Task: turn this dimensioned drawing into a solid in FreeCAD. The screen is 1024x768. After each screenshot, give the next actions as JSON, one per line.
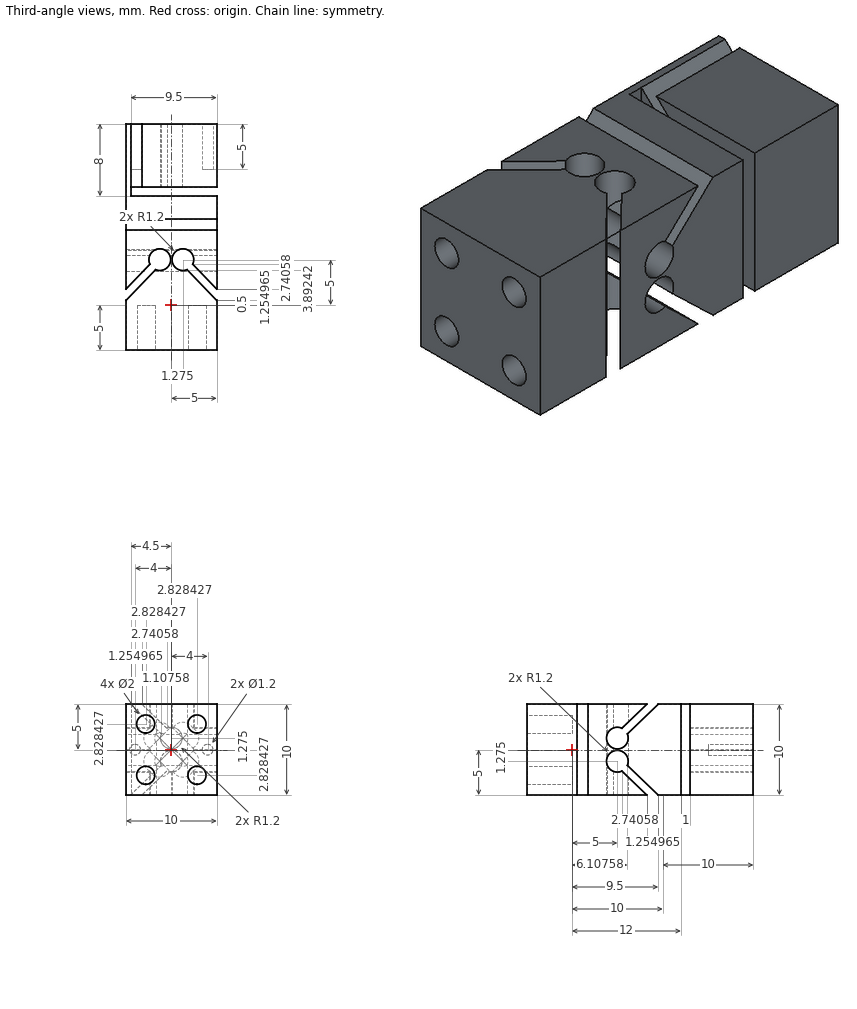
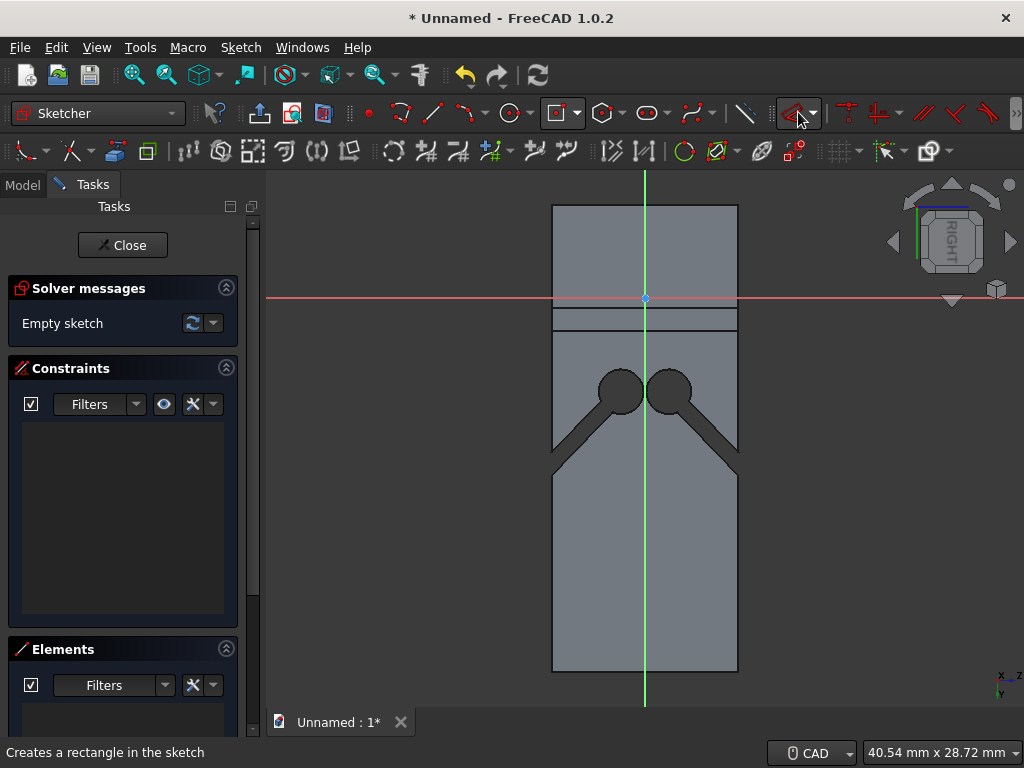
{"action": "scroll", "coordinate": [784, 382], "scroll_direction": "up", "scroll_amount": 2}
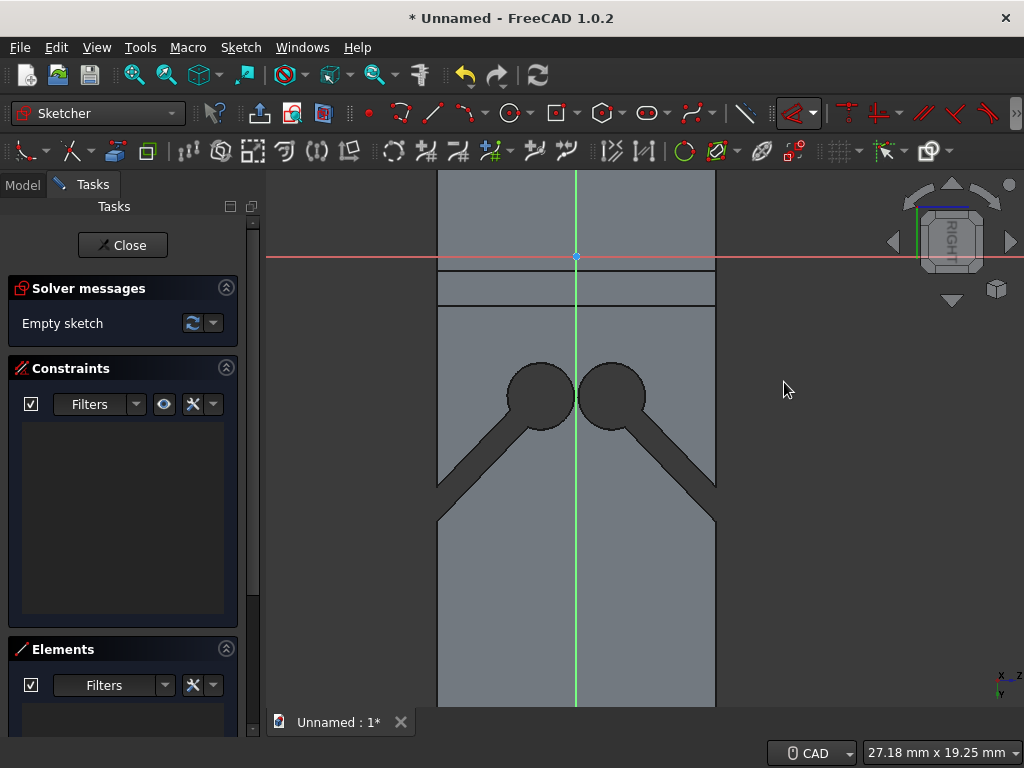
{"action": "left_click", "coordinate": [580, 114]}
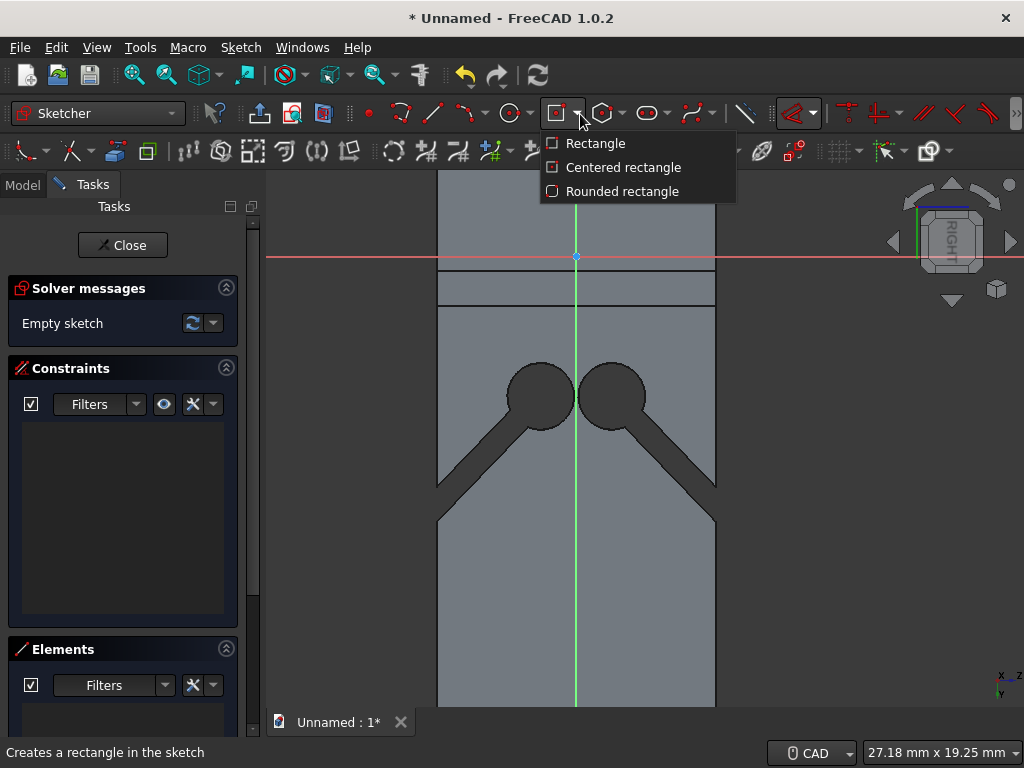
{"action": "left_click", "coordinate": [638, 143]}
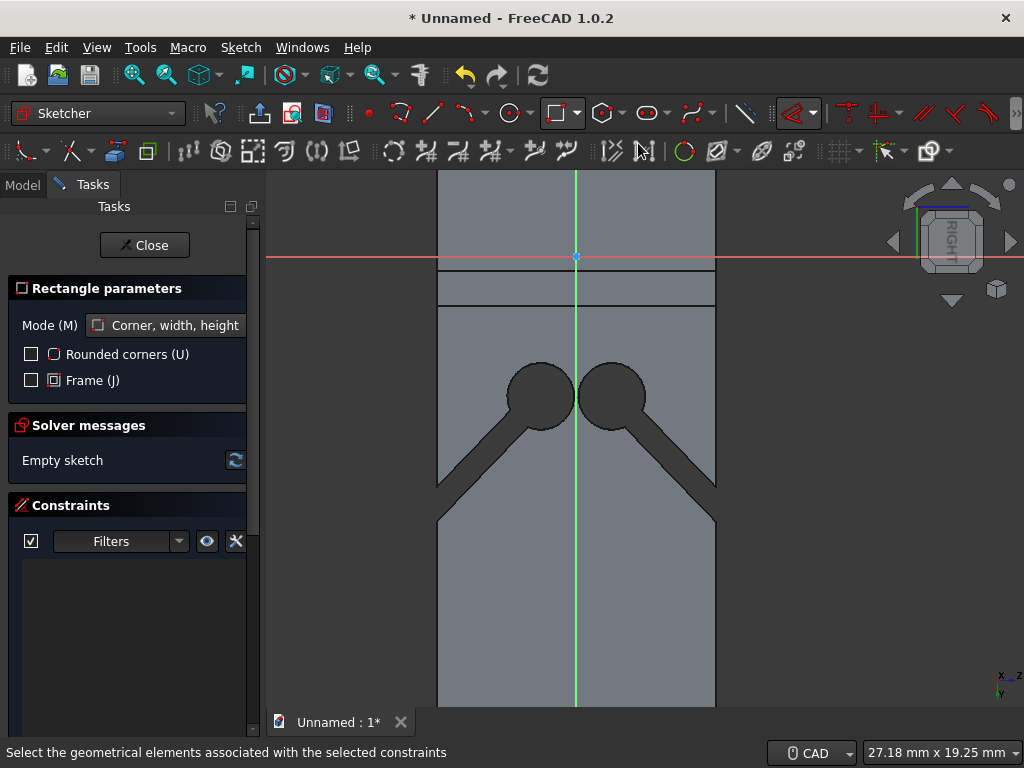
{"action": "left_click", "coordinate": [437, 592]}
{"action": "left_click", "coordinate": [716, 619]}
{"action": "key", "text": "Escape"}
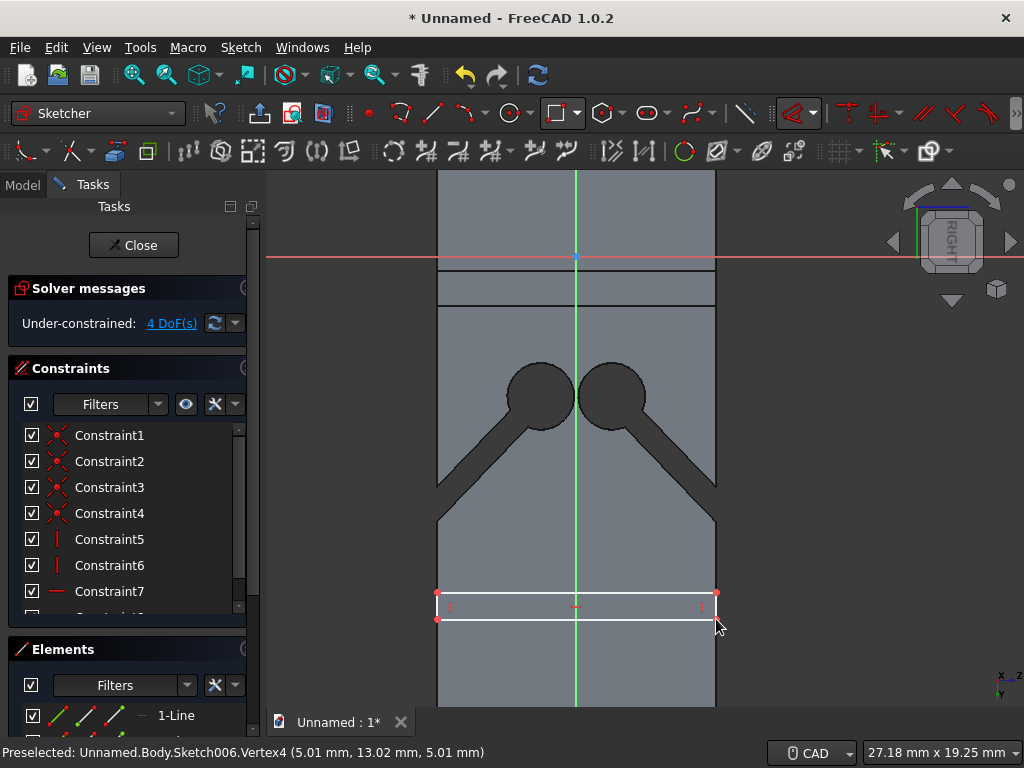
{"action": "scroll", "coordinate": [437, 604], "scroll_direction": "up", "scroll_amount": 2}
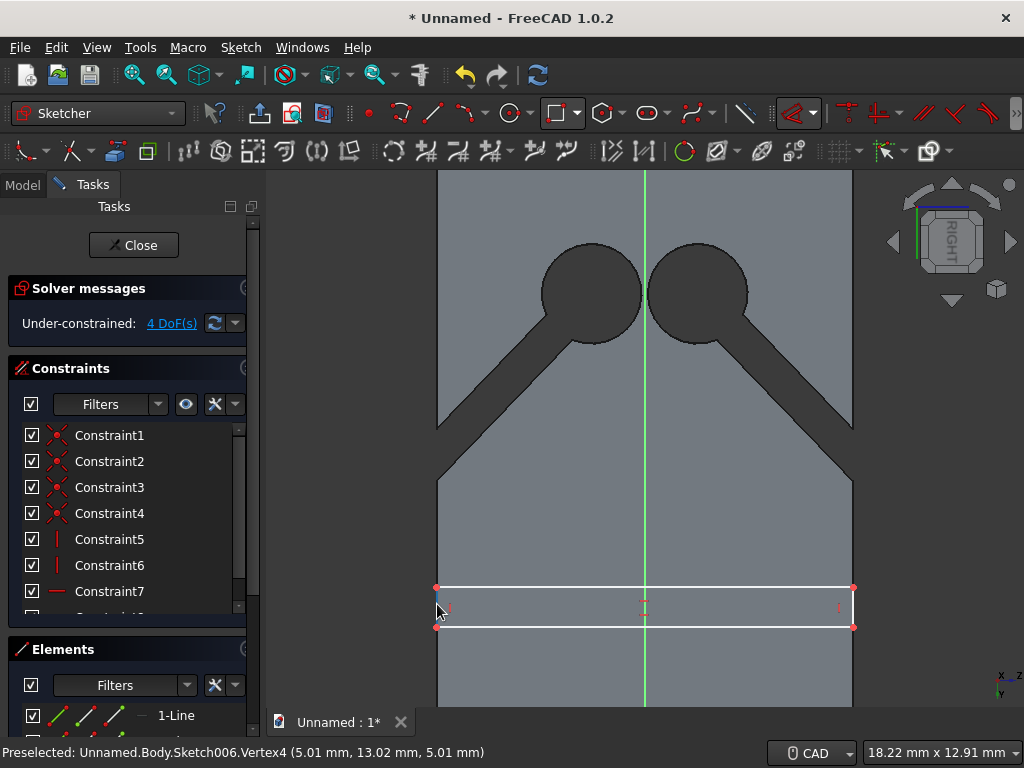
{"action": "left_click", "coordinate": [437, 603]}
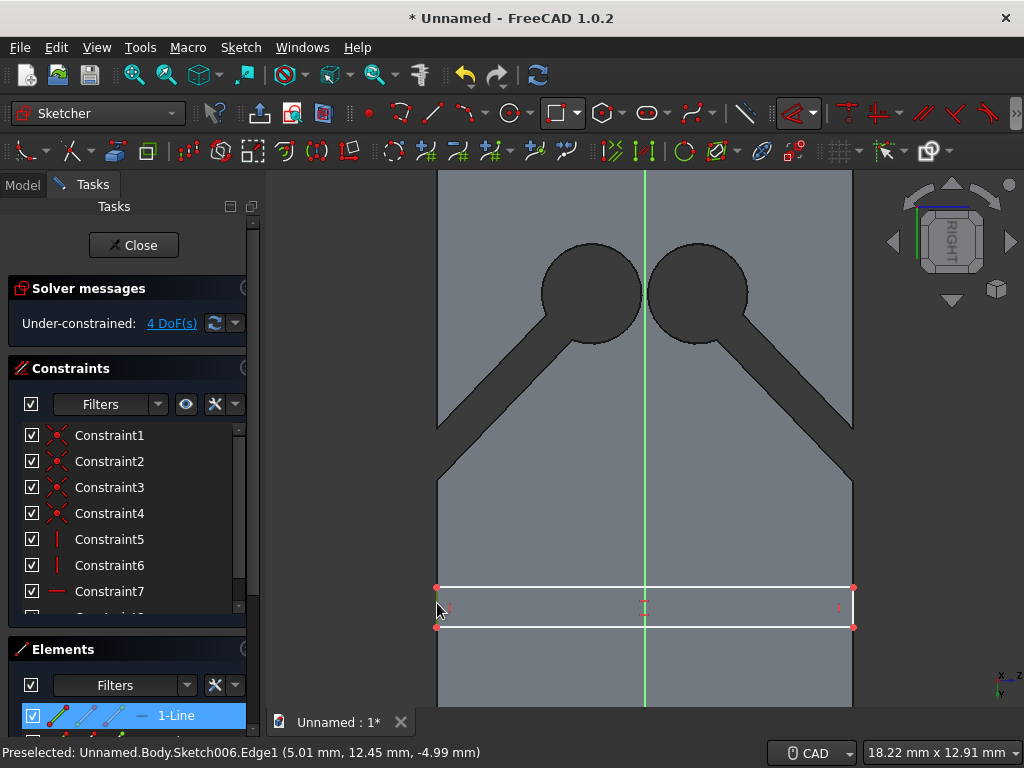
{"action": "key", "text": "i"}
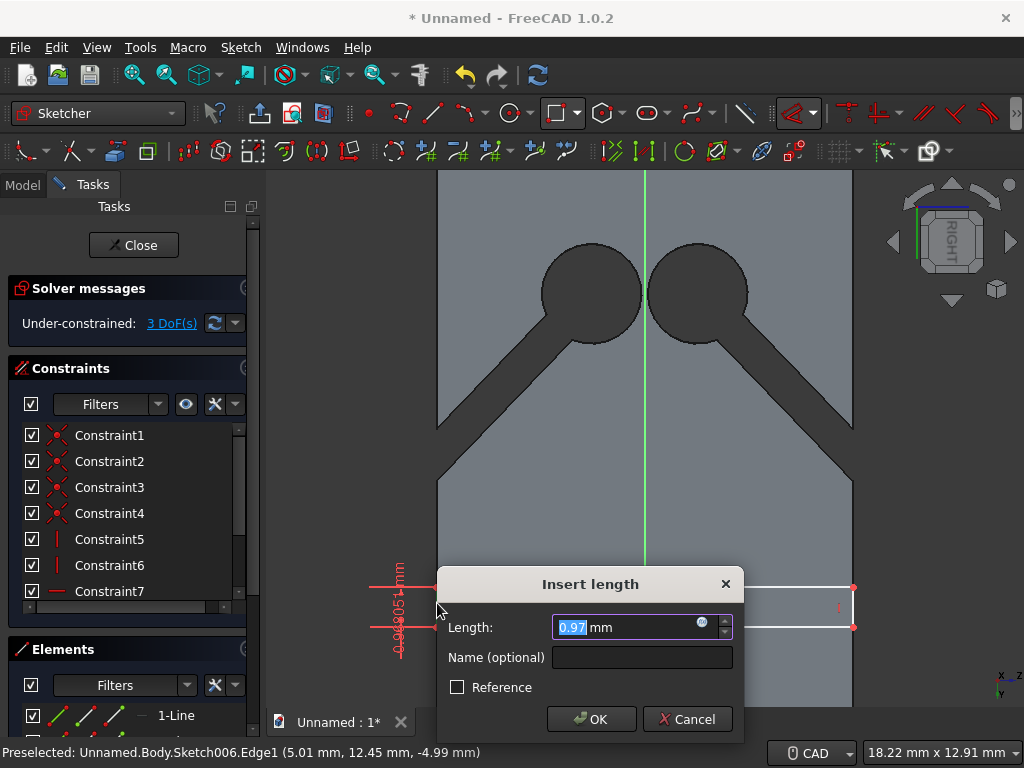
{"action": "type", "text": "1"}
{"action": "key", "text": "Return"}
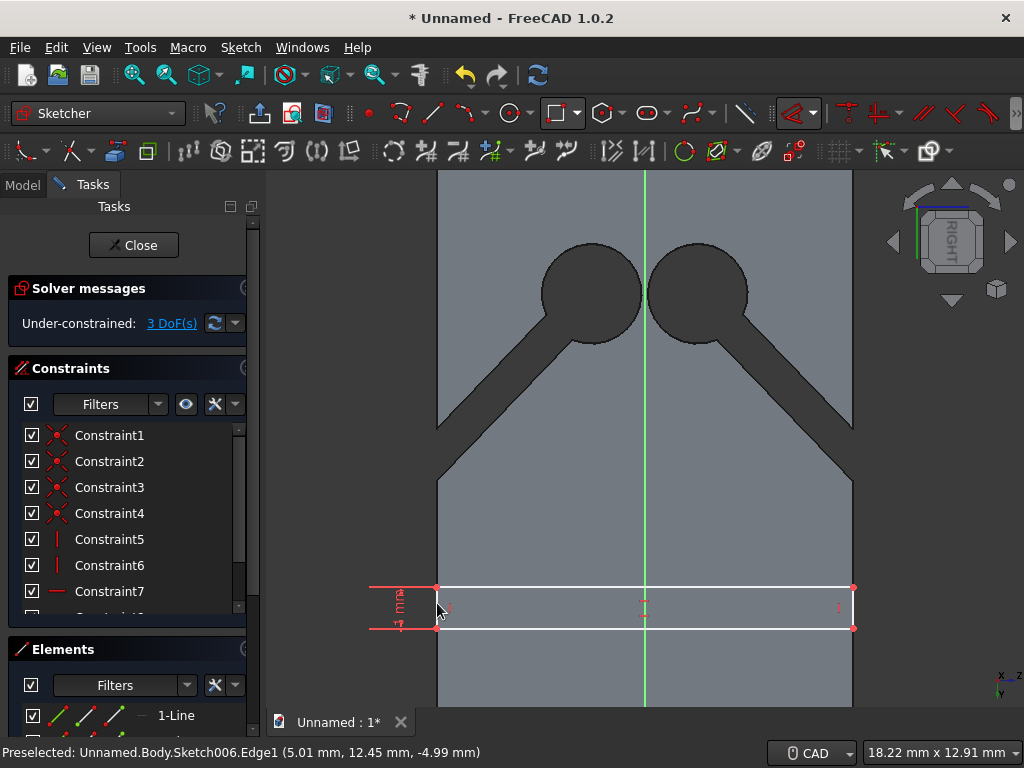
{"action": "left_click", "coordinate": [562, 629]}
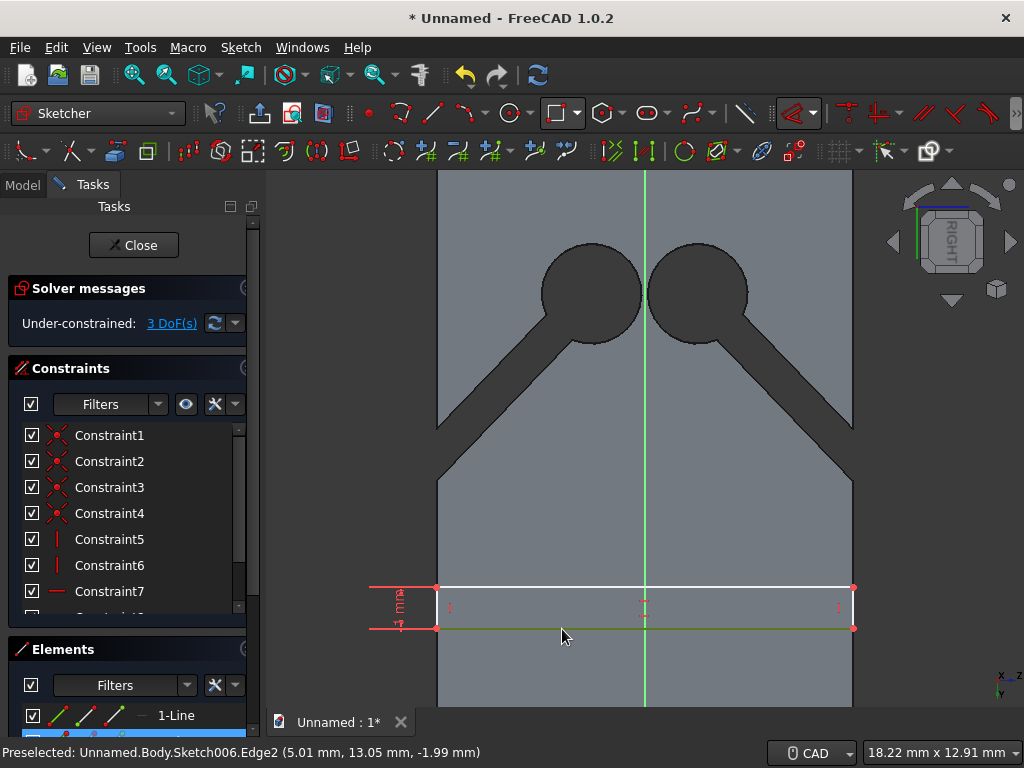
{"action": "left_click", "coordinate": [816, 114]}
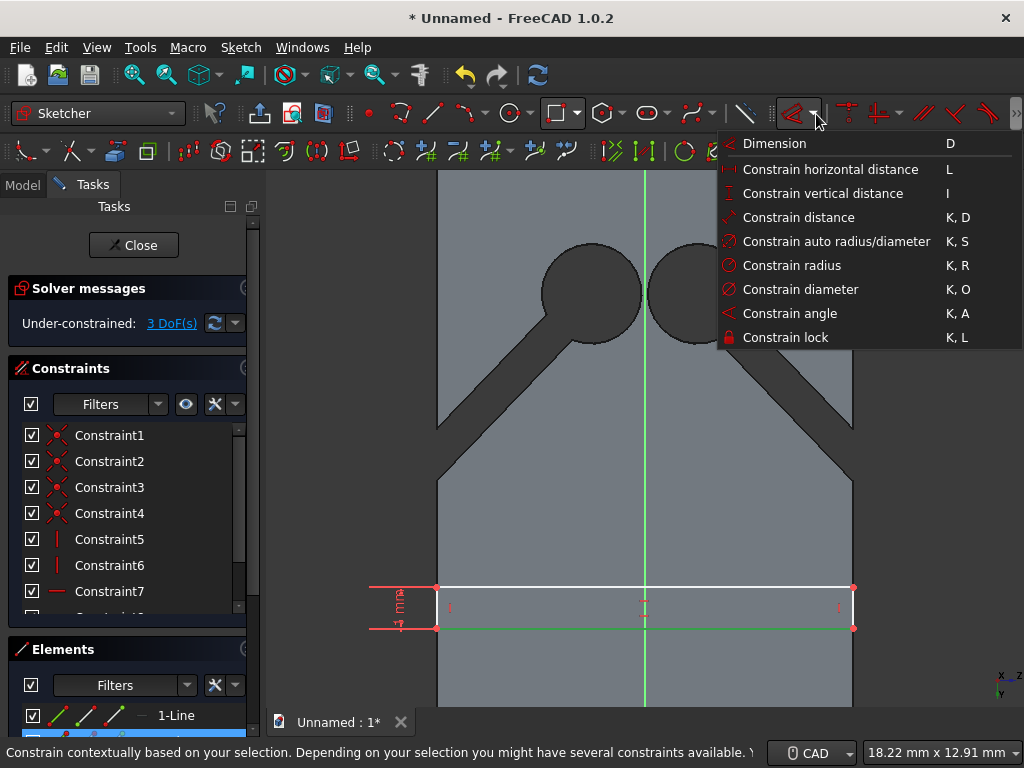
{"action": "left_click", "coordinate": [870, 169]}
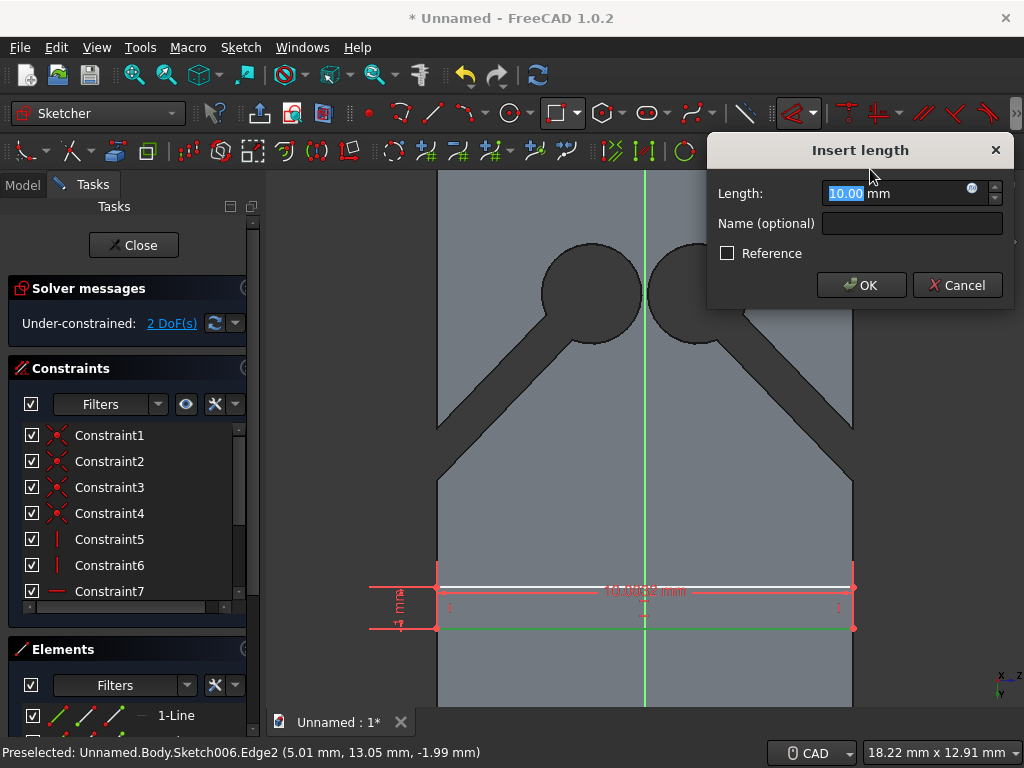
{"action": "type", "text": "10"}
{"action": "key", "text": "Return"}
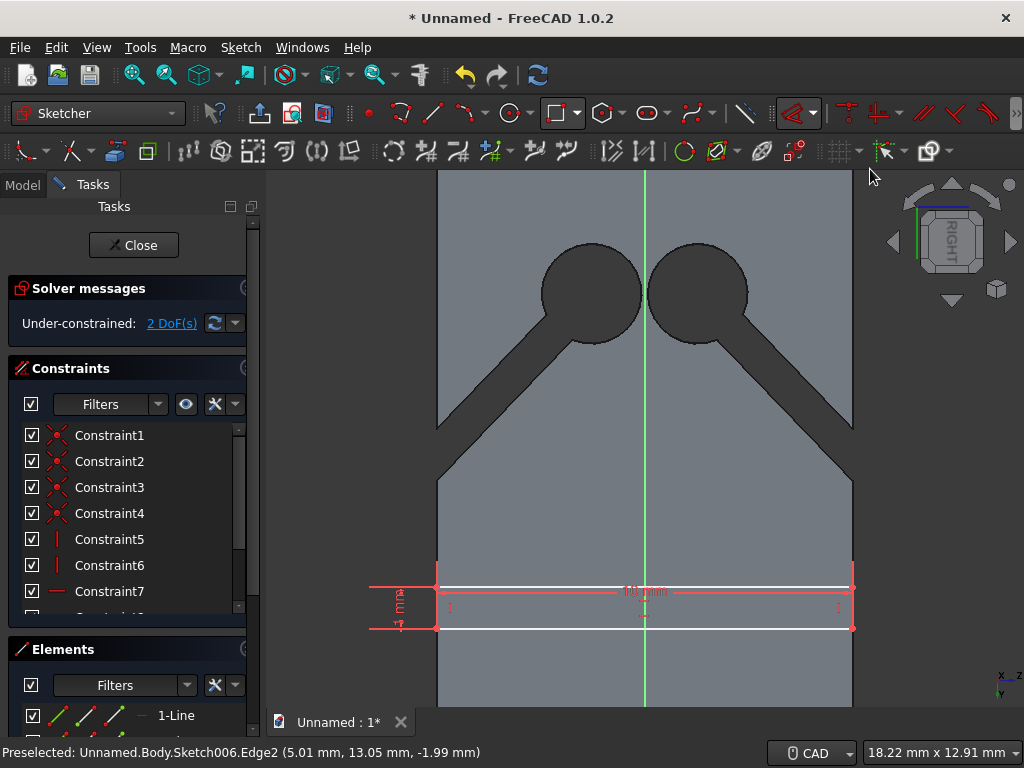
{"action": "left_click", "coordinate": [437, 587]}